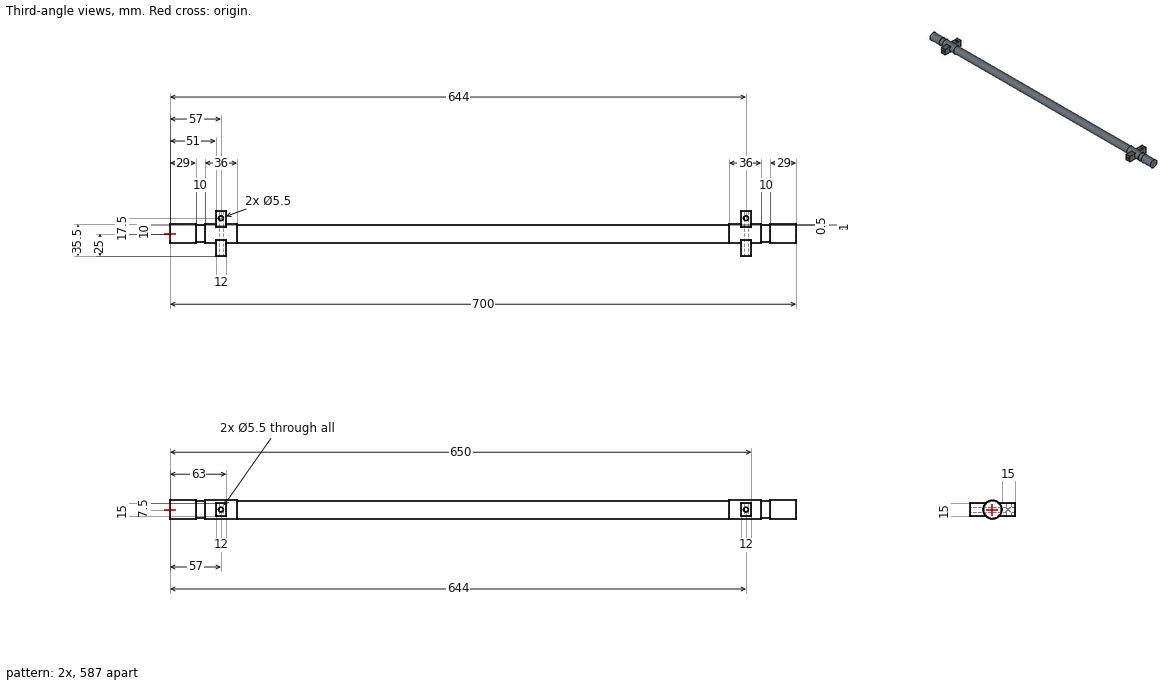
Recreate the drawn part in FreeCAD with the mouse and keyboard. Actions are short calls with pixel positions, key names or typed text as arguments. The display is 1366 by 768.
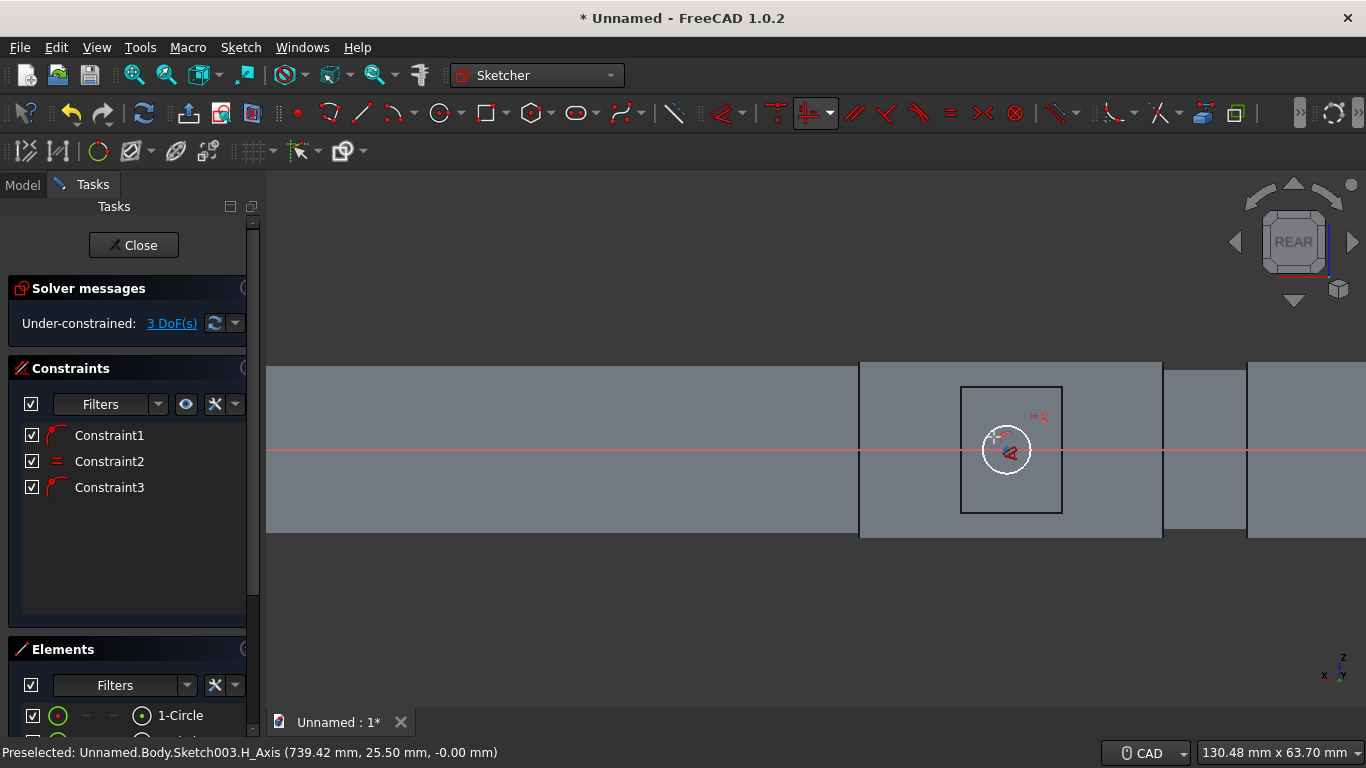
click(990, 433)
click(967, 410)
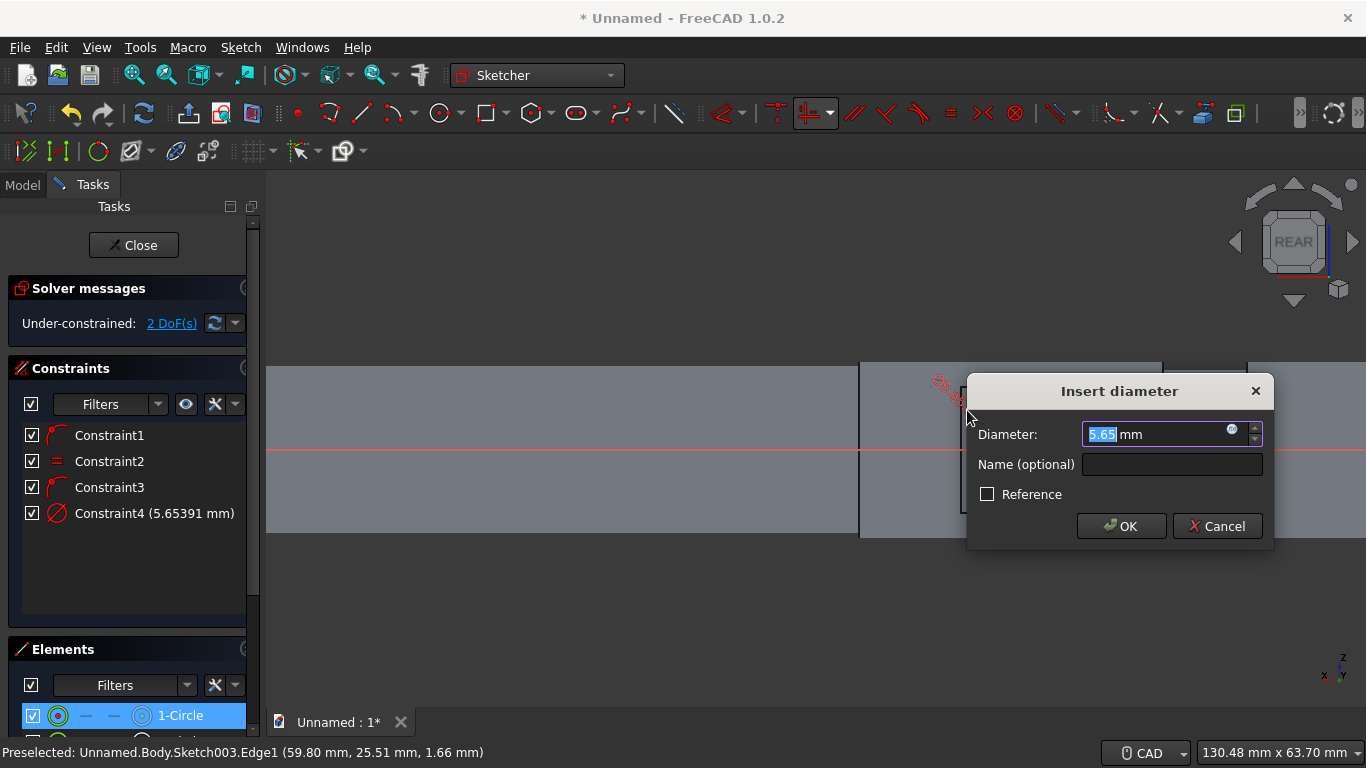
text(5.5)
key(Return)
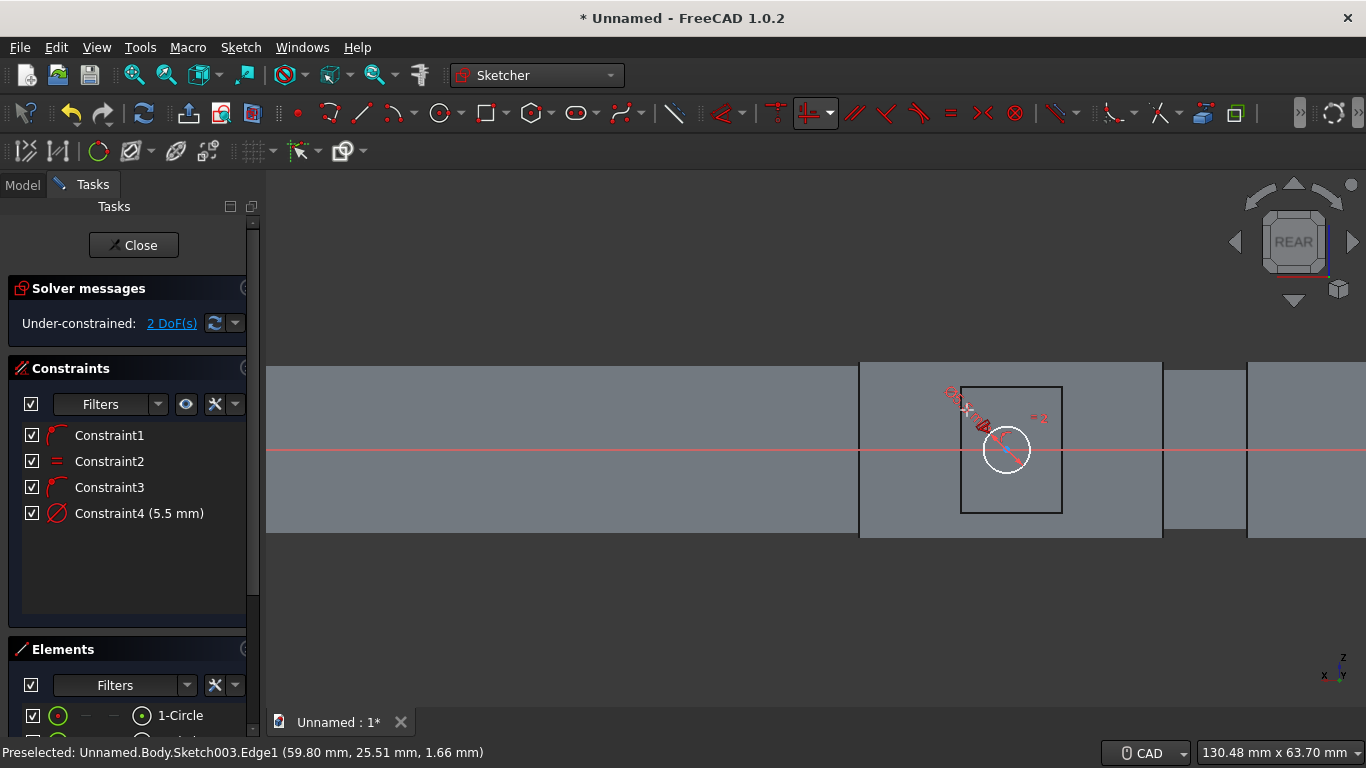
scroll(994, 437, down, 11)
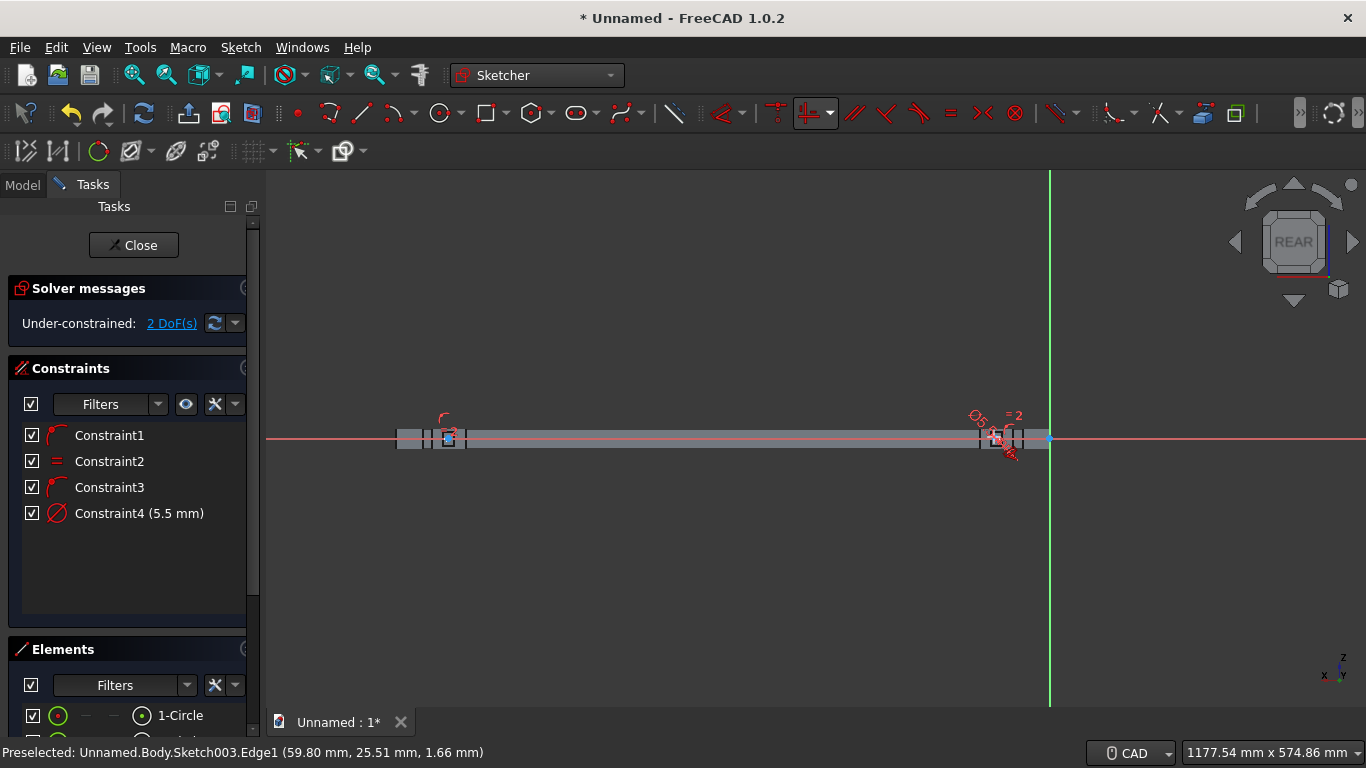
click(996, 439)
click(1023, 473)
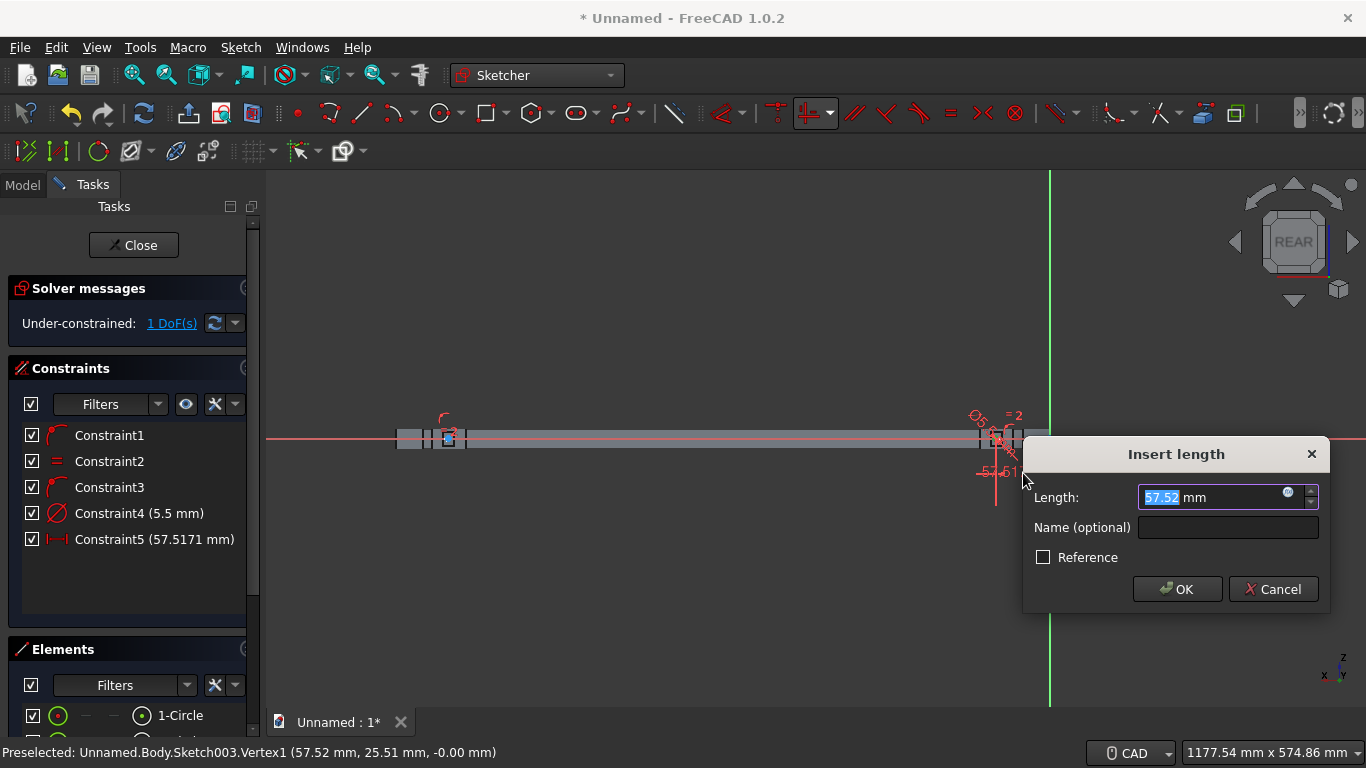
text(57)
key(Return)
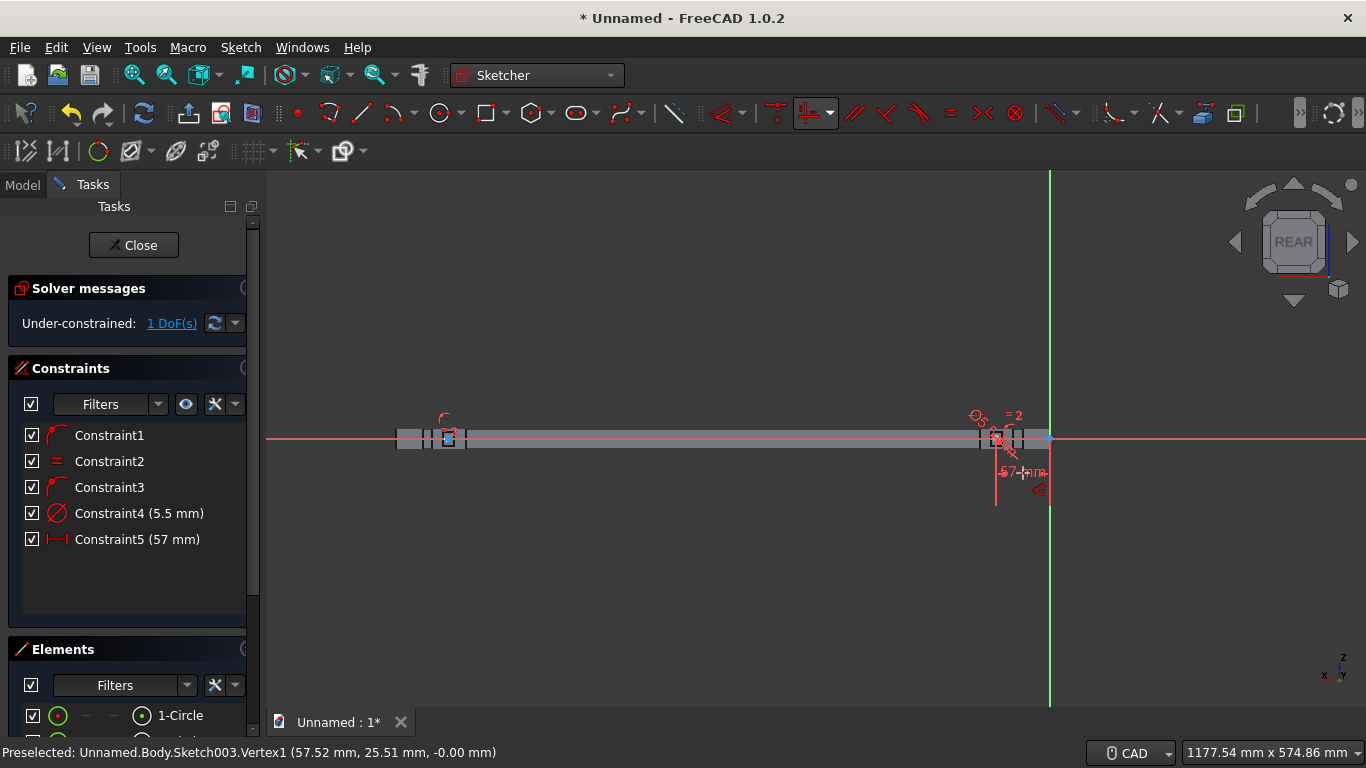
click(448, 439)
click(749, 473)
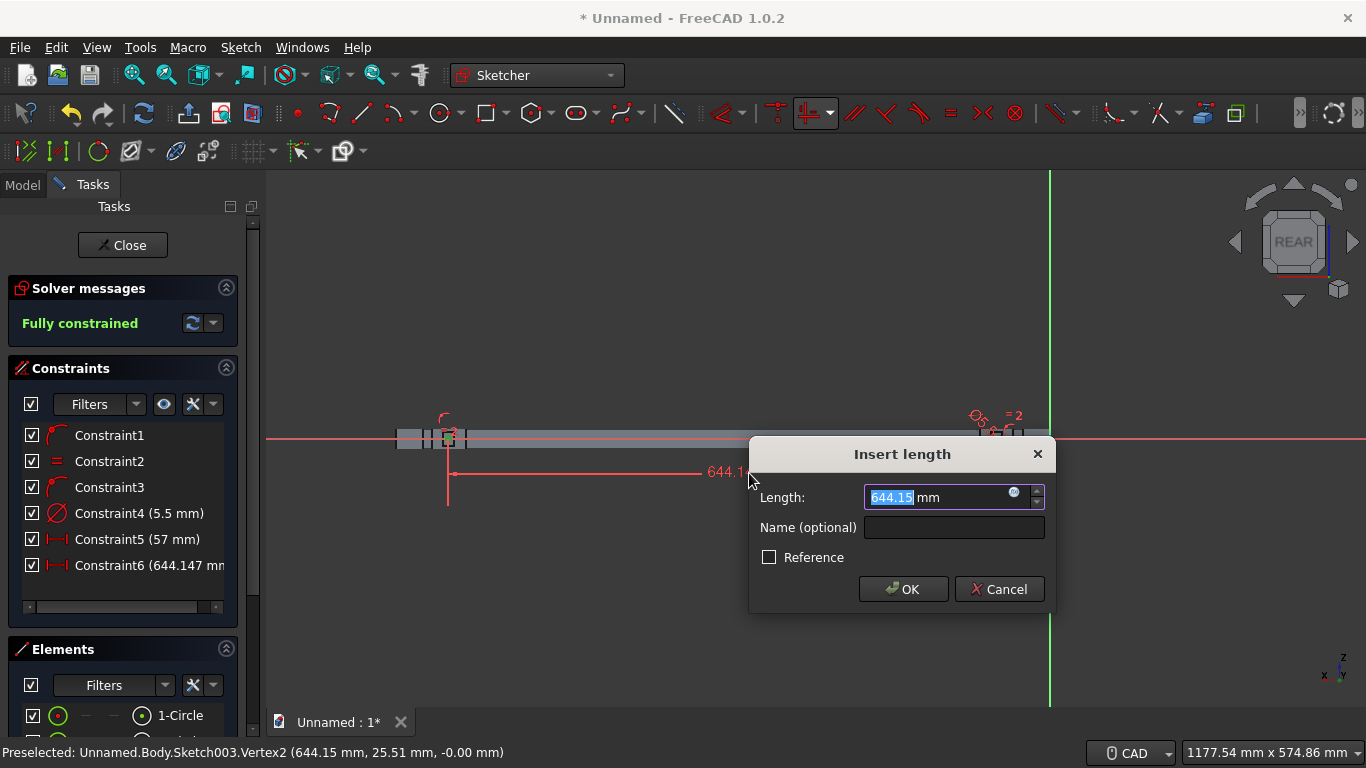
text(644)
key(Return)
key(Escape)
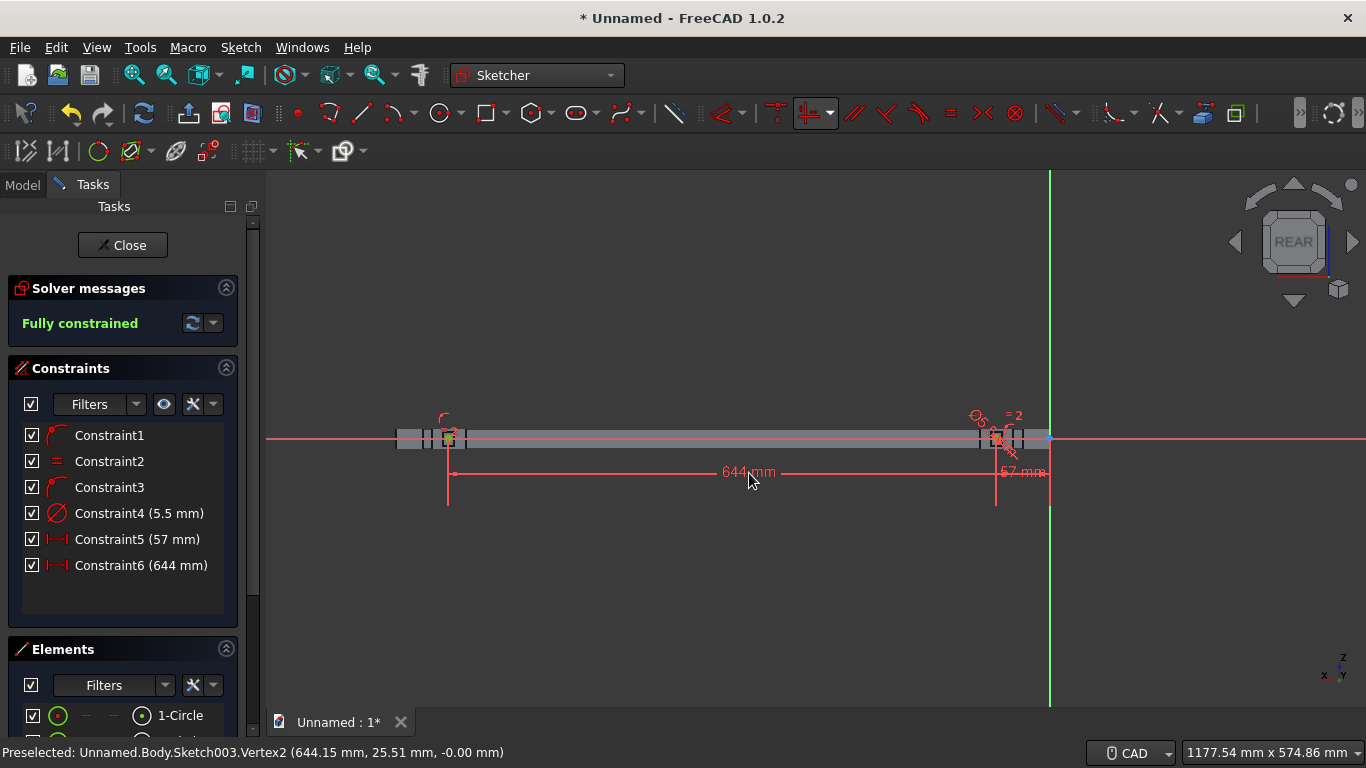
click(123, 245)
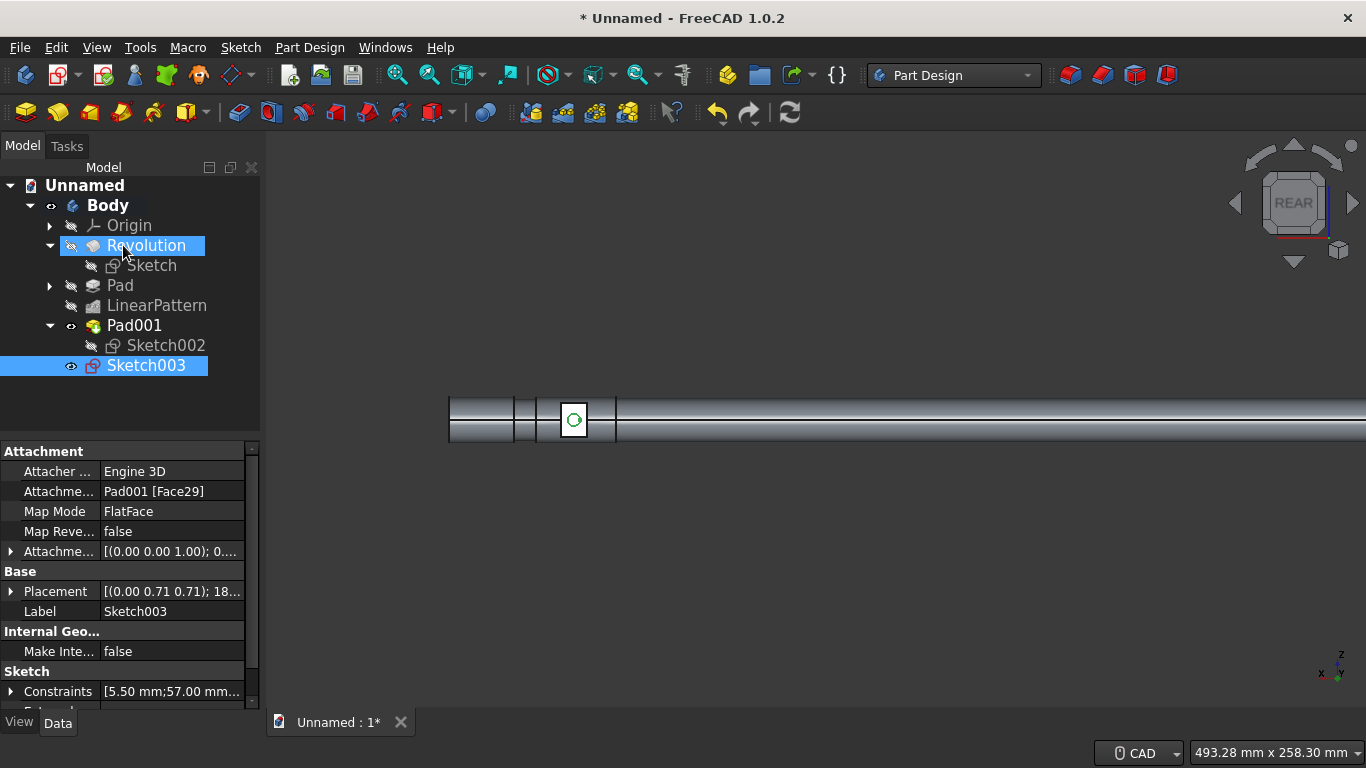
click(272, 112)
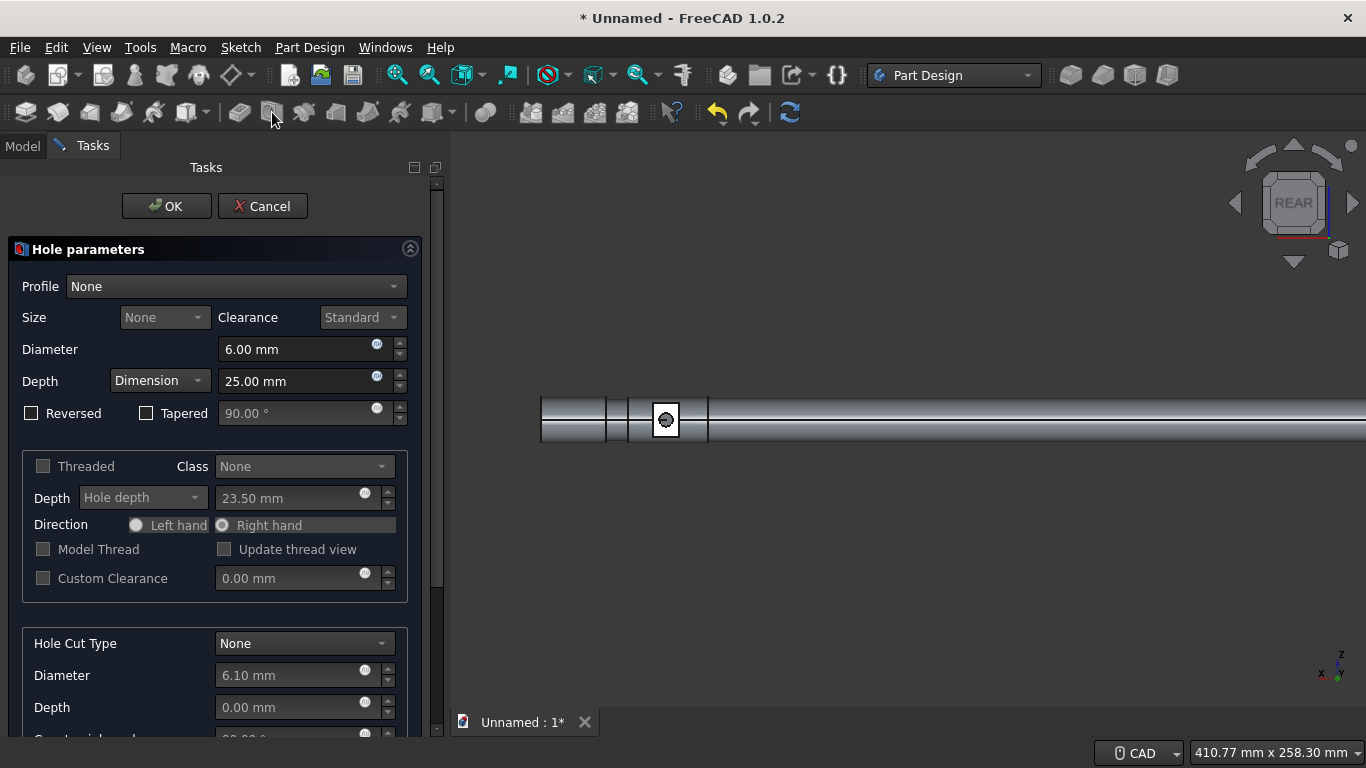
triple_click(305, 349)